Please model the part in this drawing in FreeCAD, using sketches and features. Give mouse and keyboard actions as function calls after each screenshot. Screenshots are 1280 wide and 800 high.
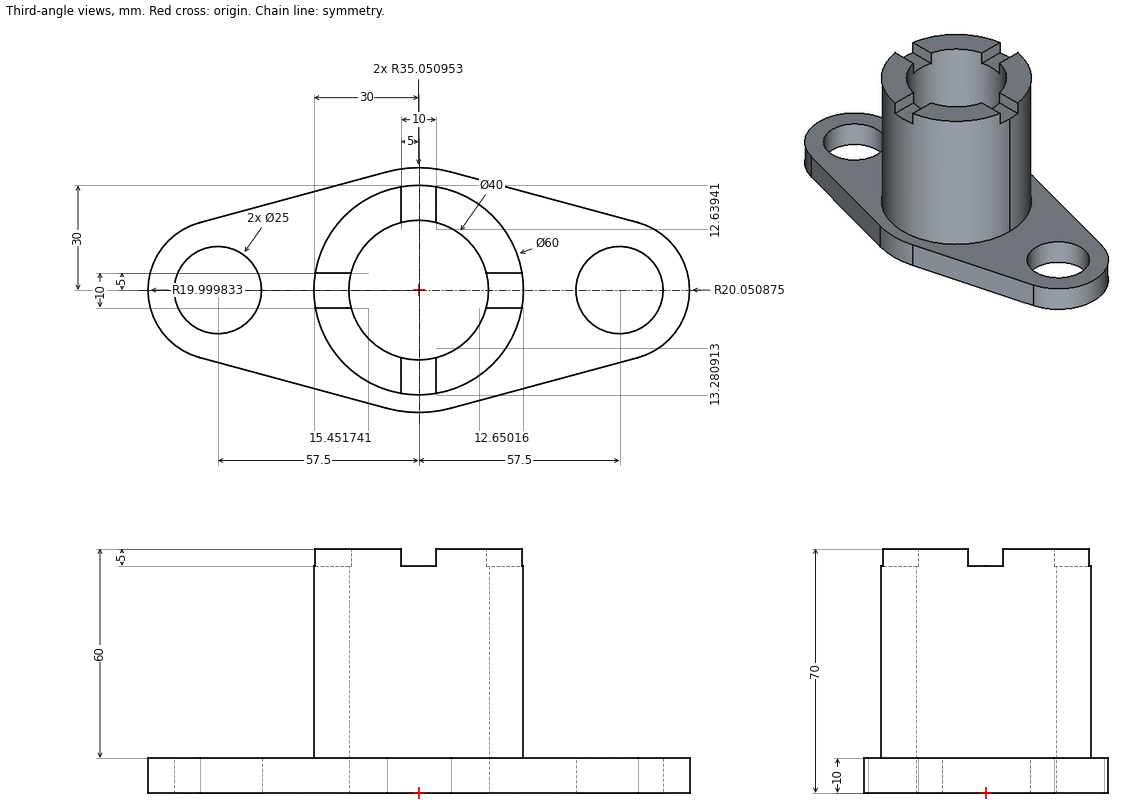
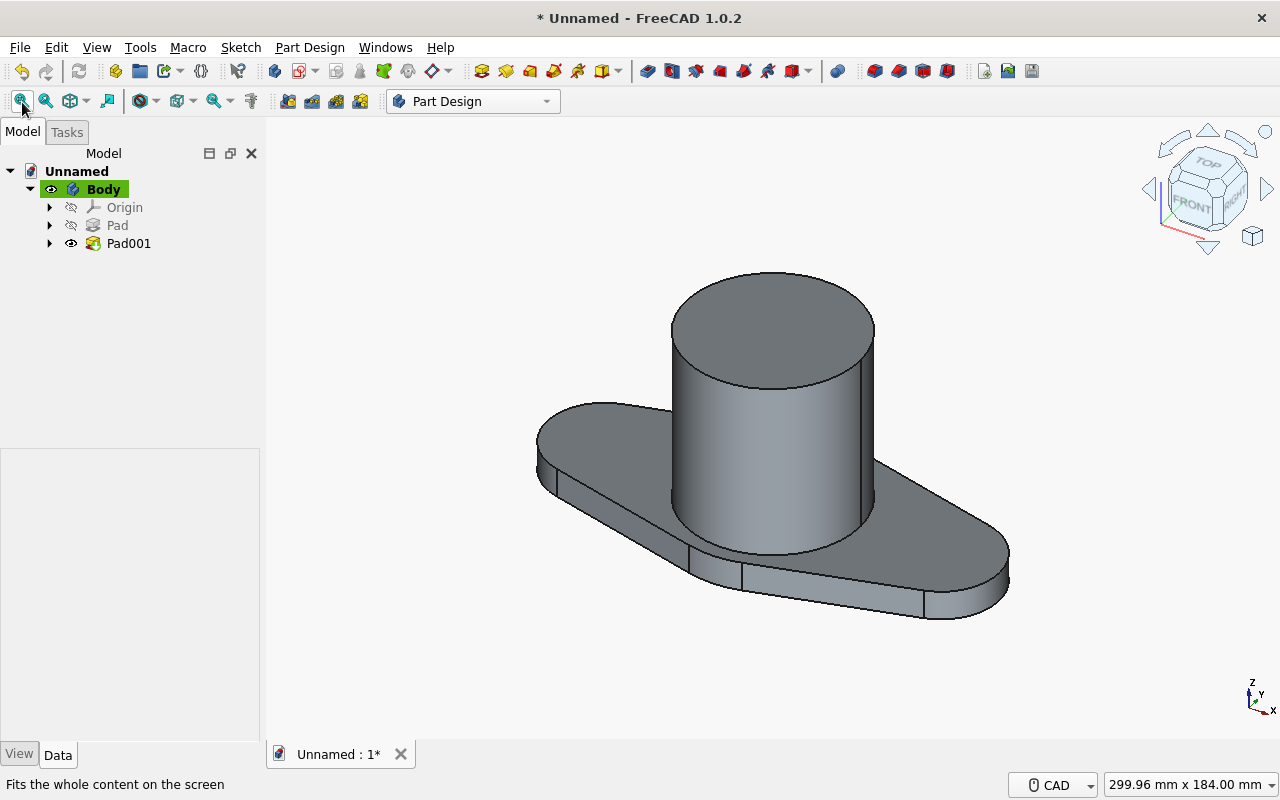
click(773, 330)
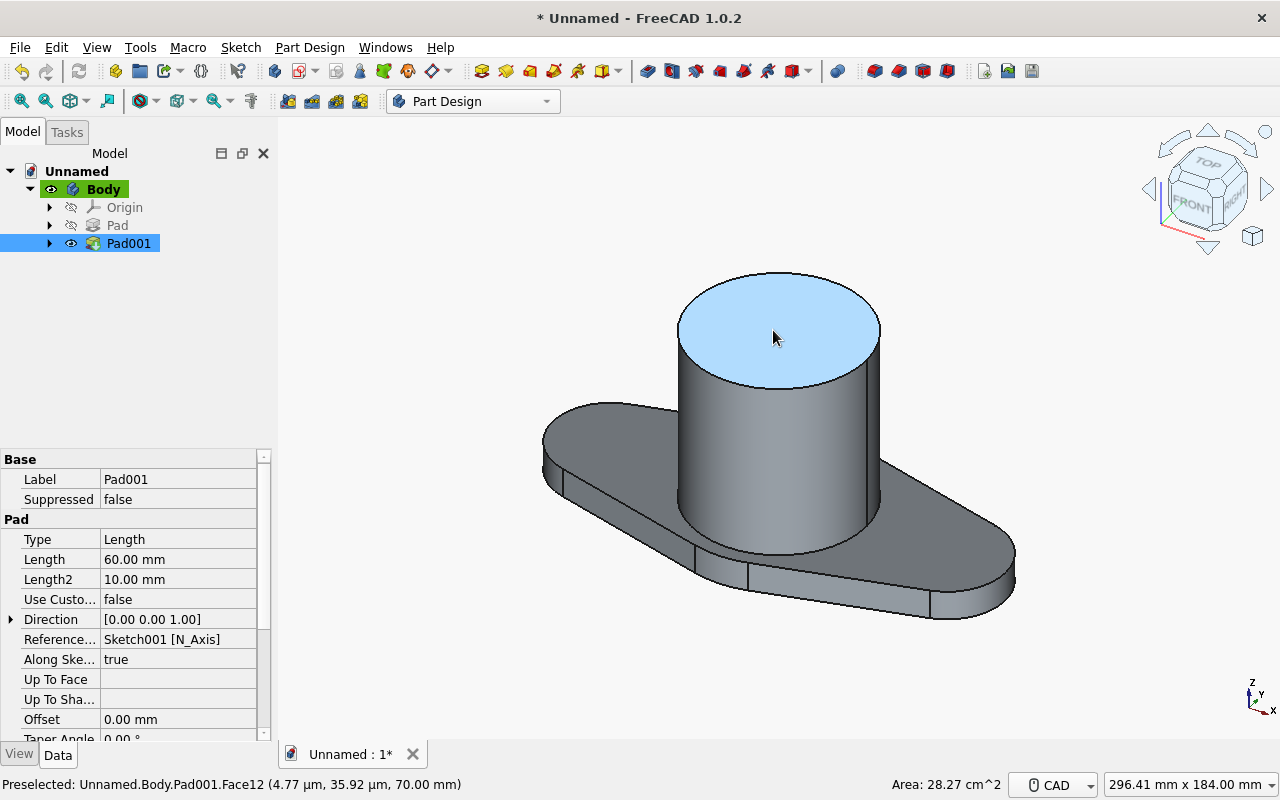
click(300, 72)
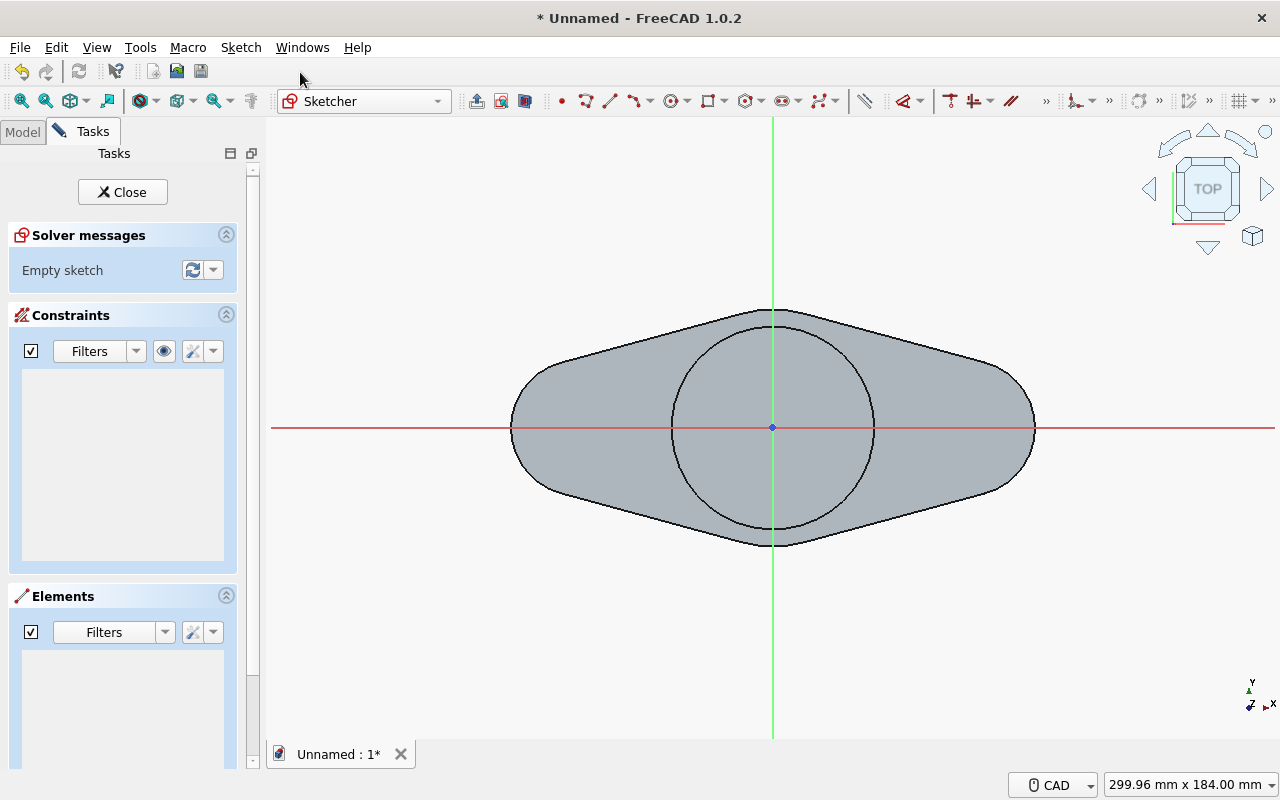
scroll(813, 428, up, 5)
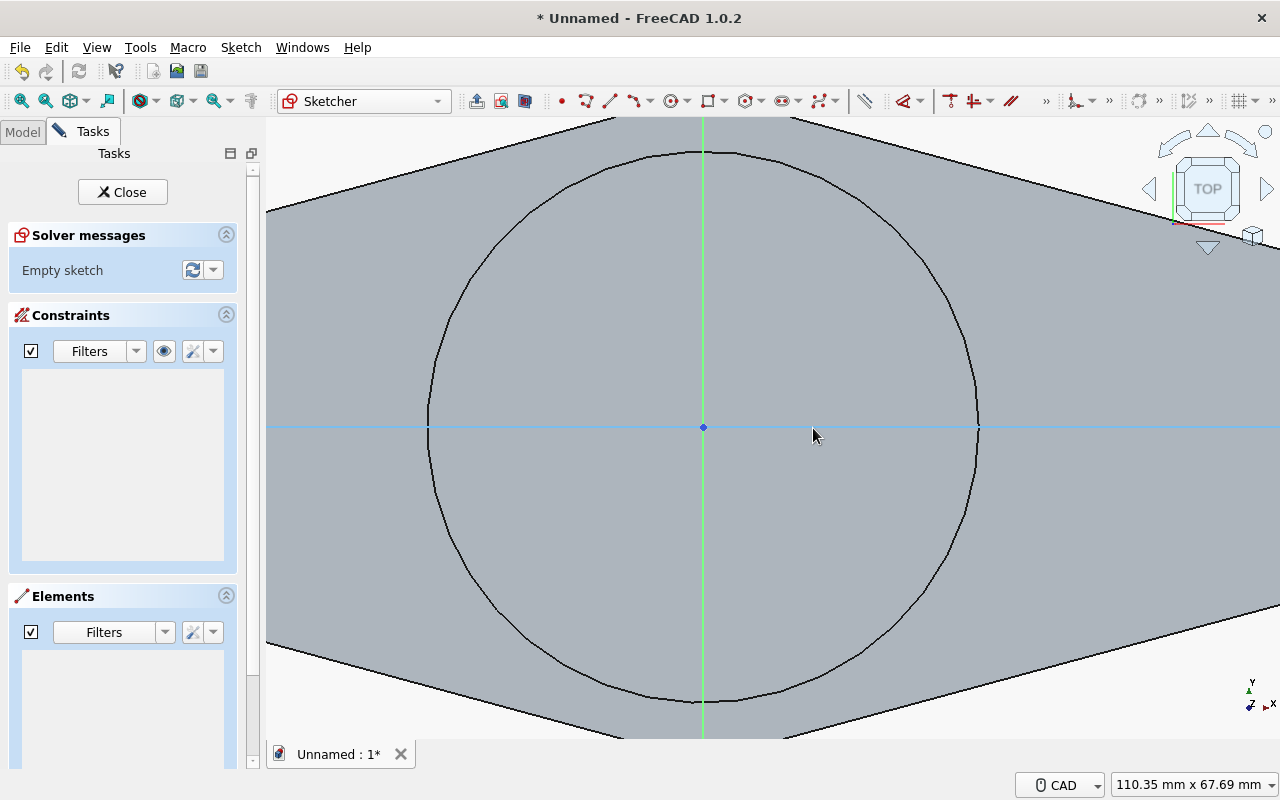
key(g)
key(c)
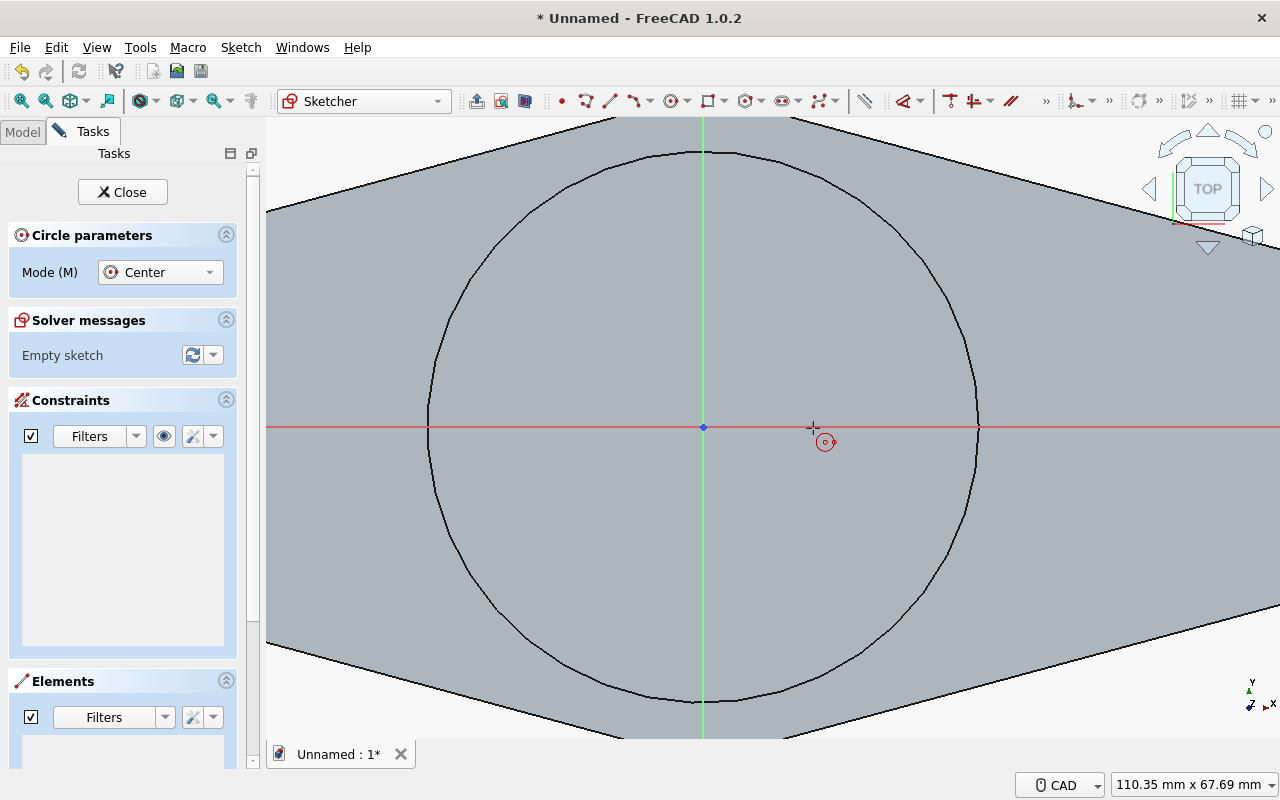
click(703, 427)
move(833, 297)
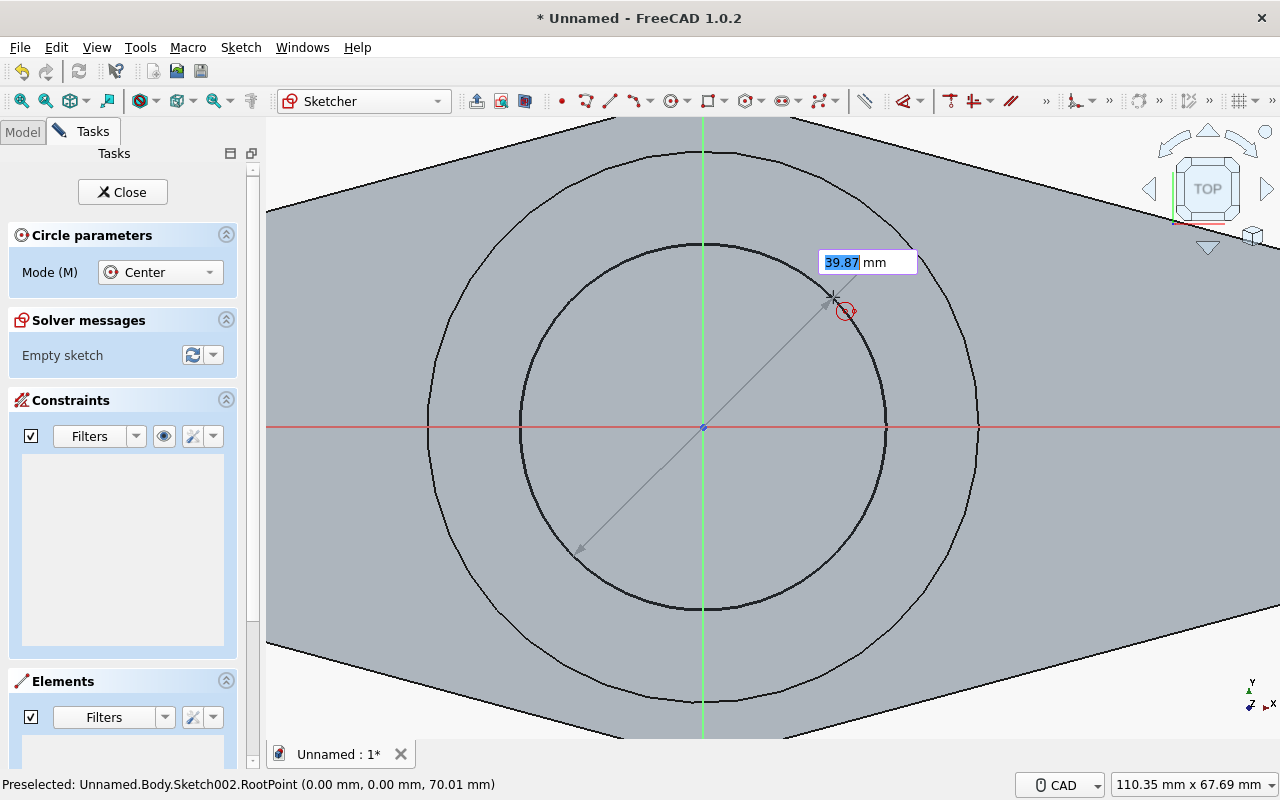
text(40)
key(Return)
key(Escape)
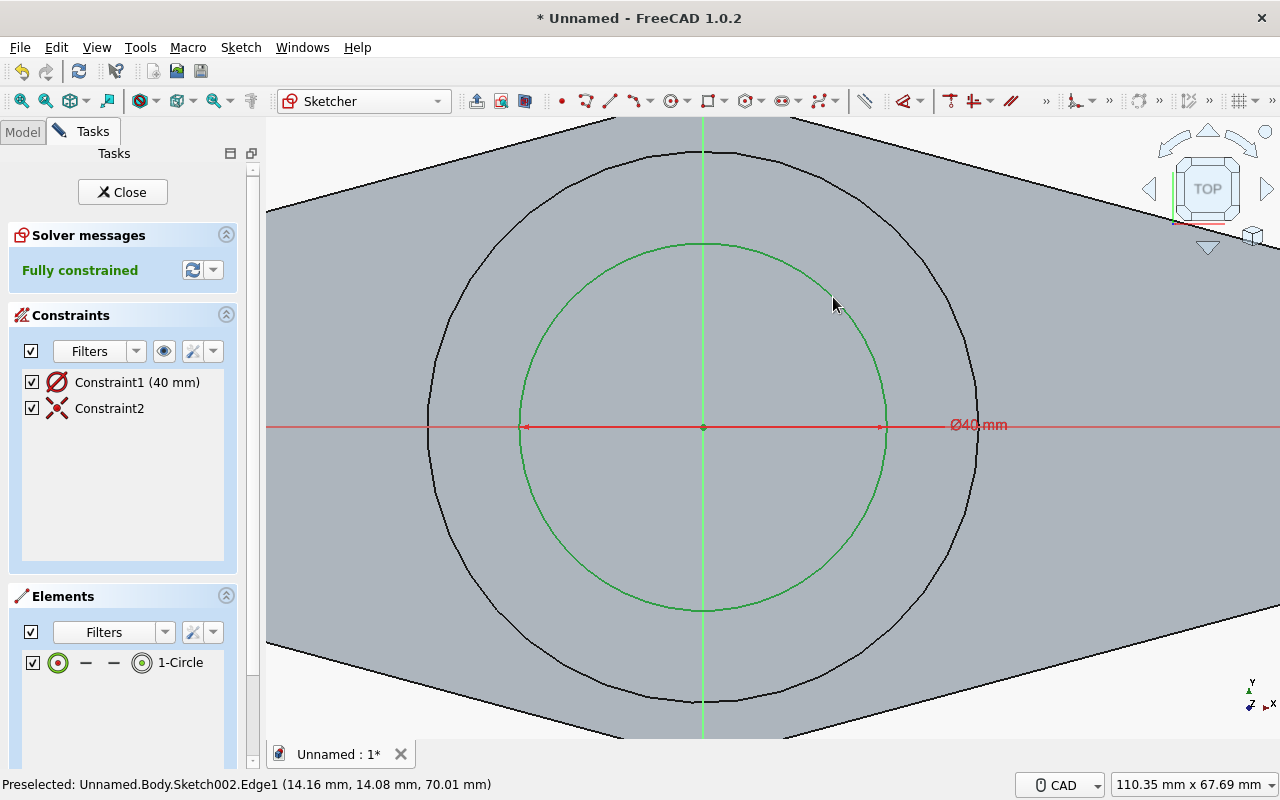
click(123, 192)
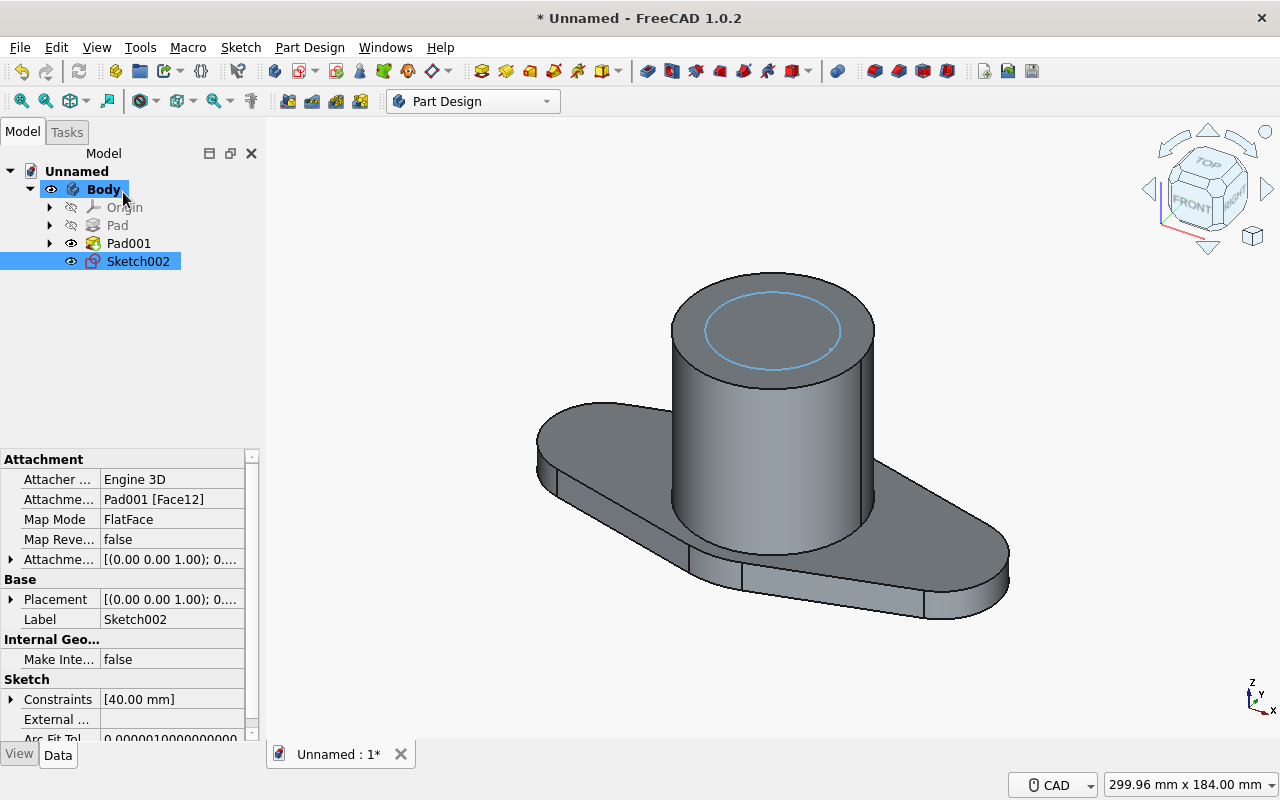
click(648, 72)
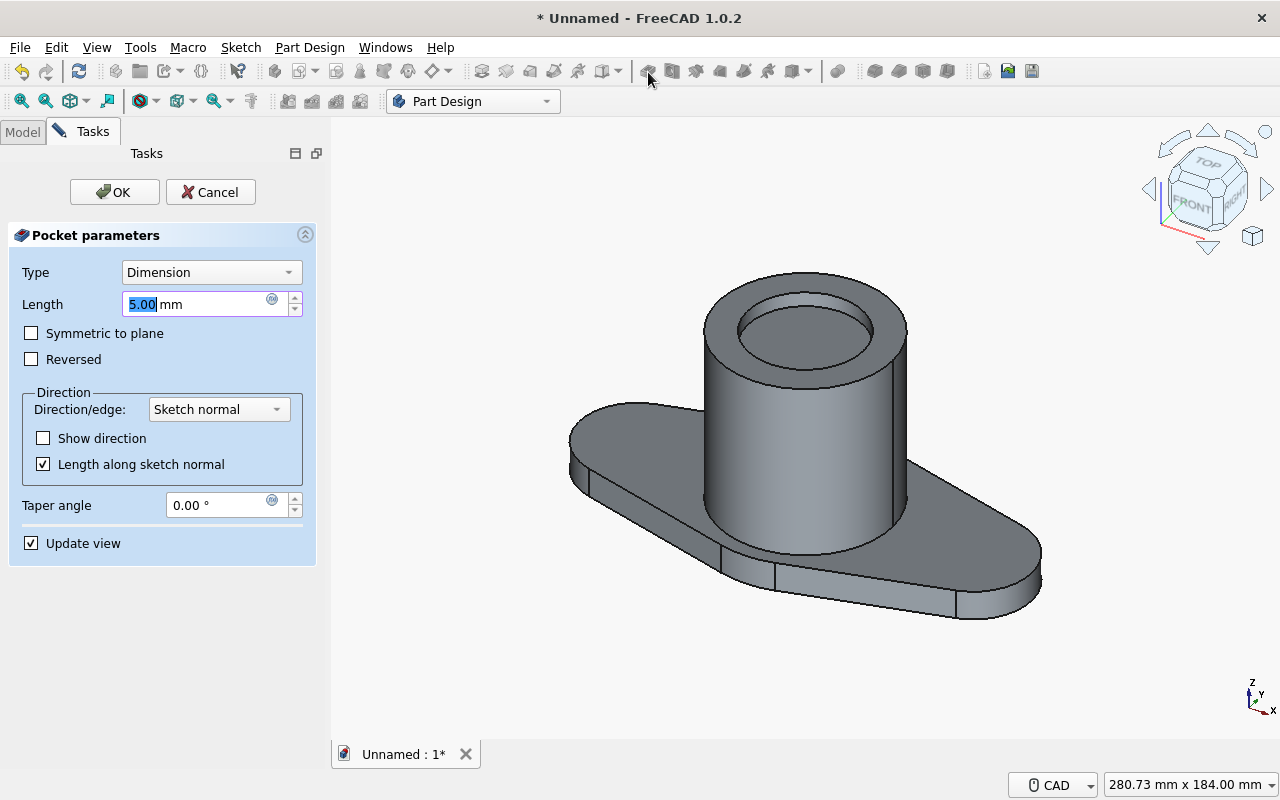
text(70)
key(Tab)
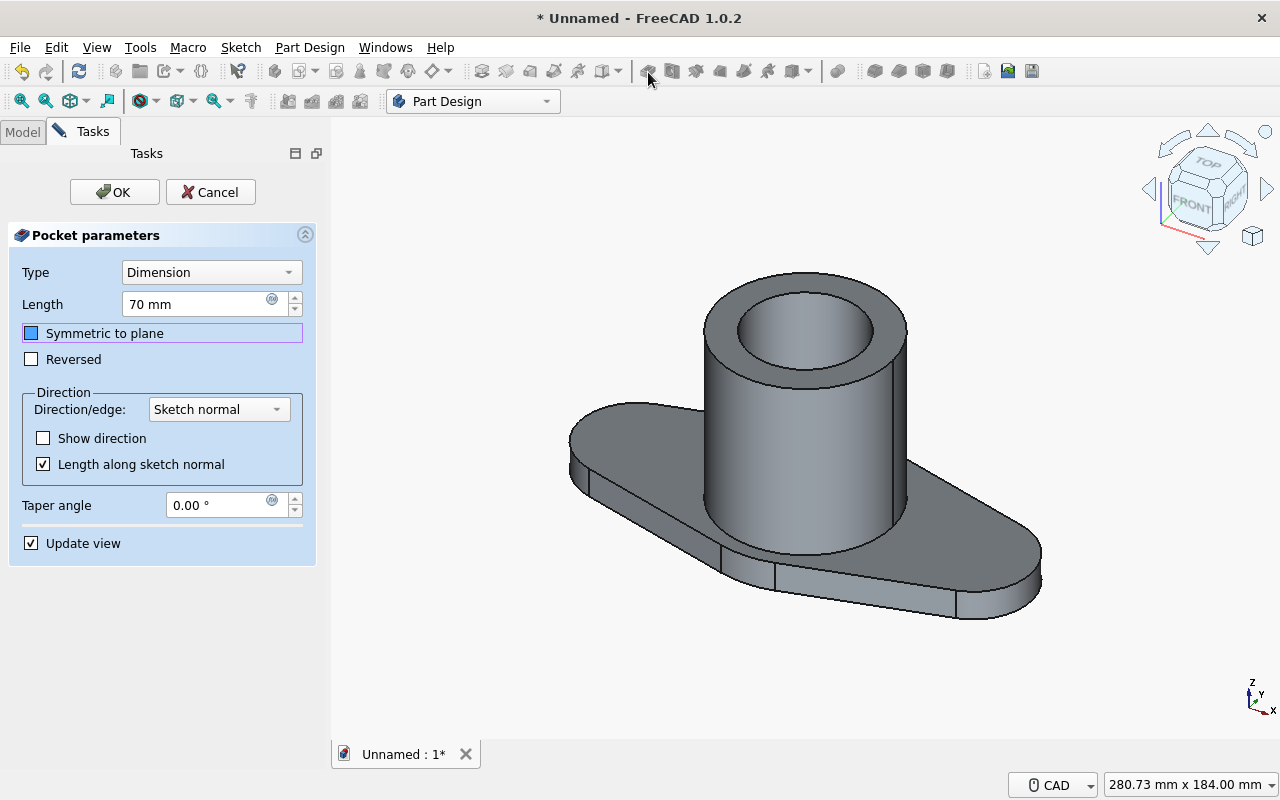
click(115, 192)